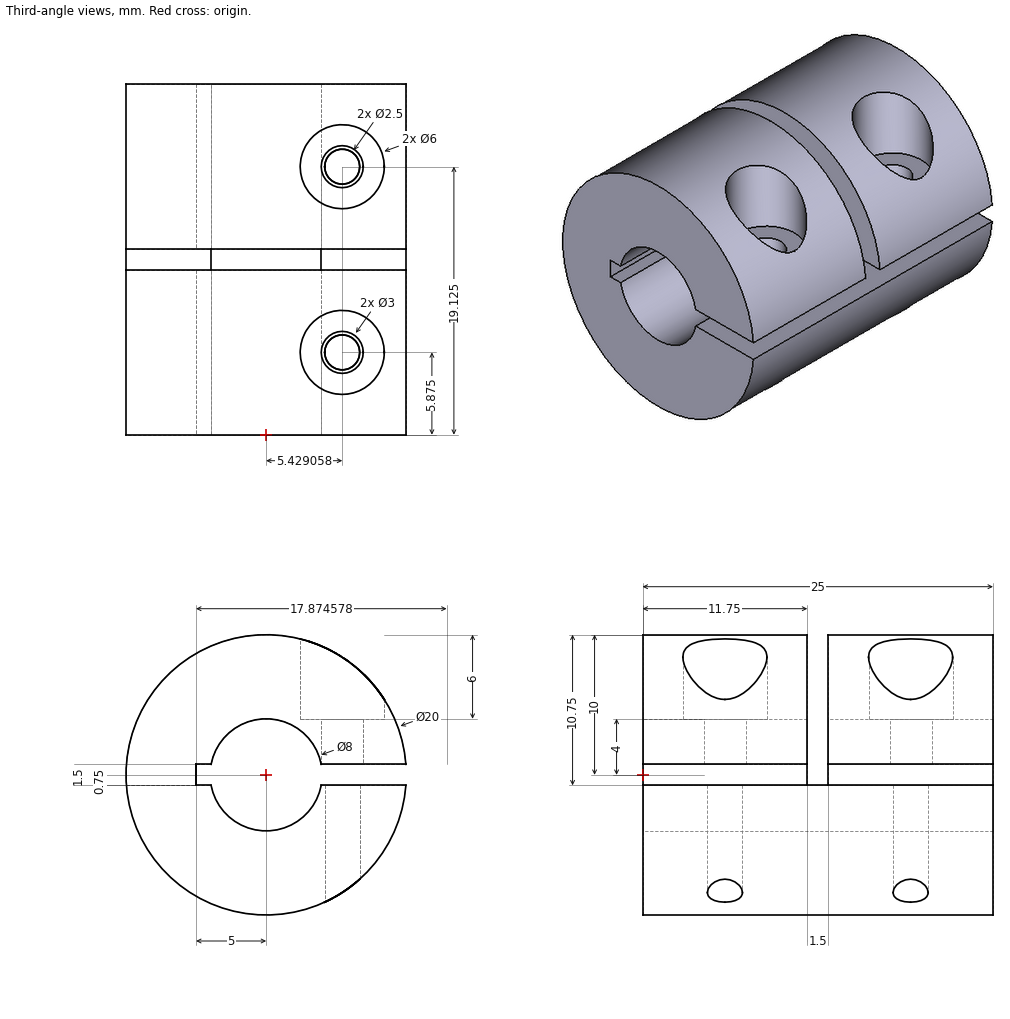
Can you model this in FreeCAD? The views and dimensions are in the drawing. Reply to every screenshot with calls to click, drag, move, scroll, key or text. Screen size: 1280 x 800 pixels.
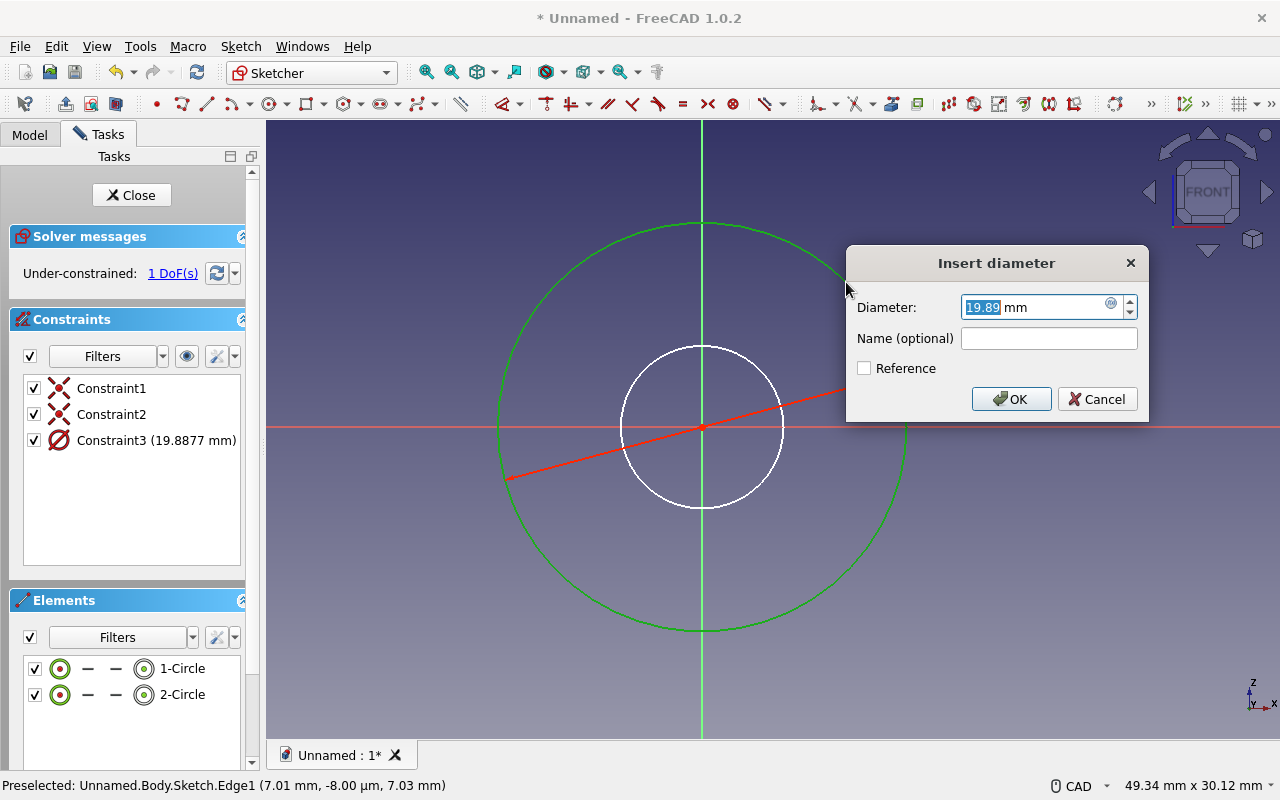
text(20)
key(Return)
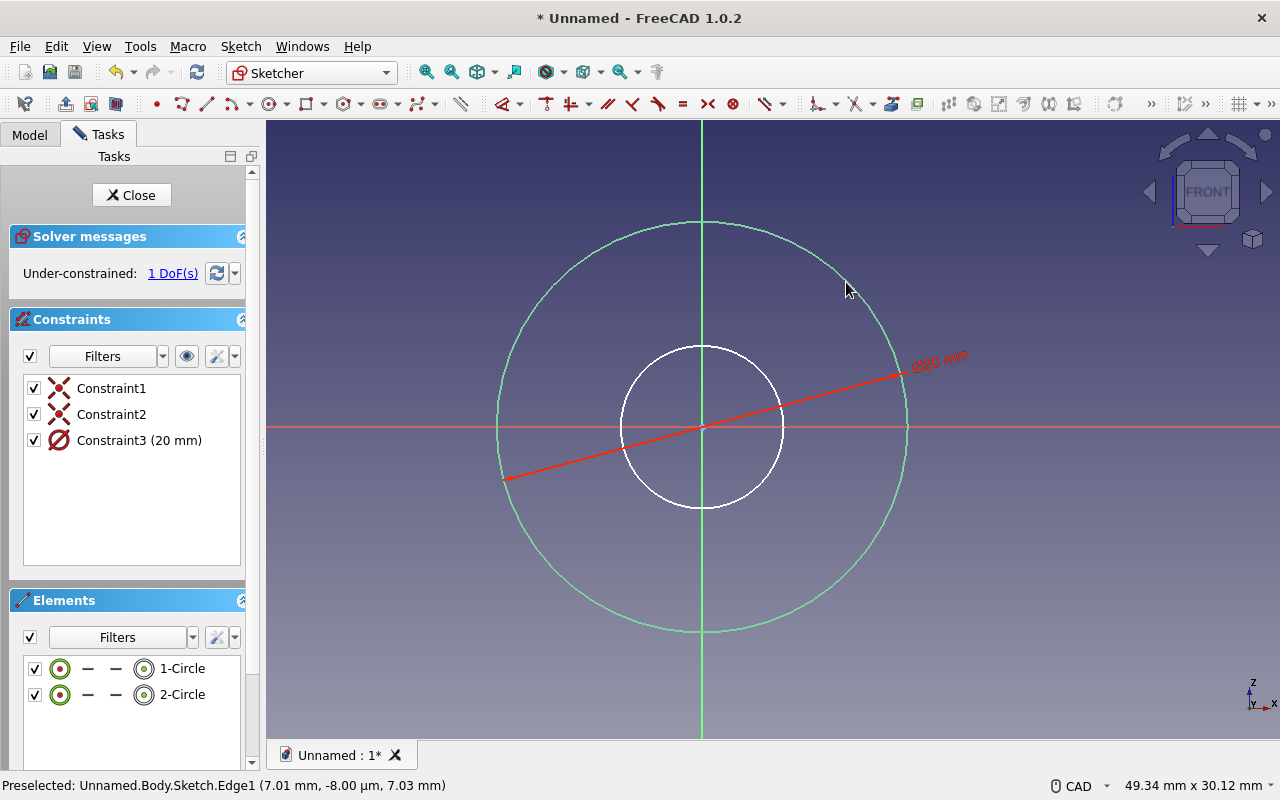
click(759, 369)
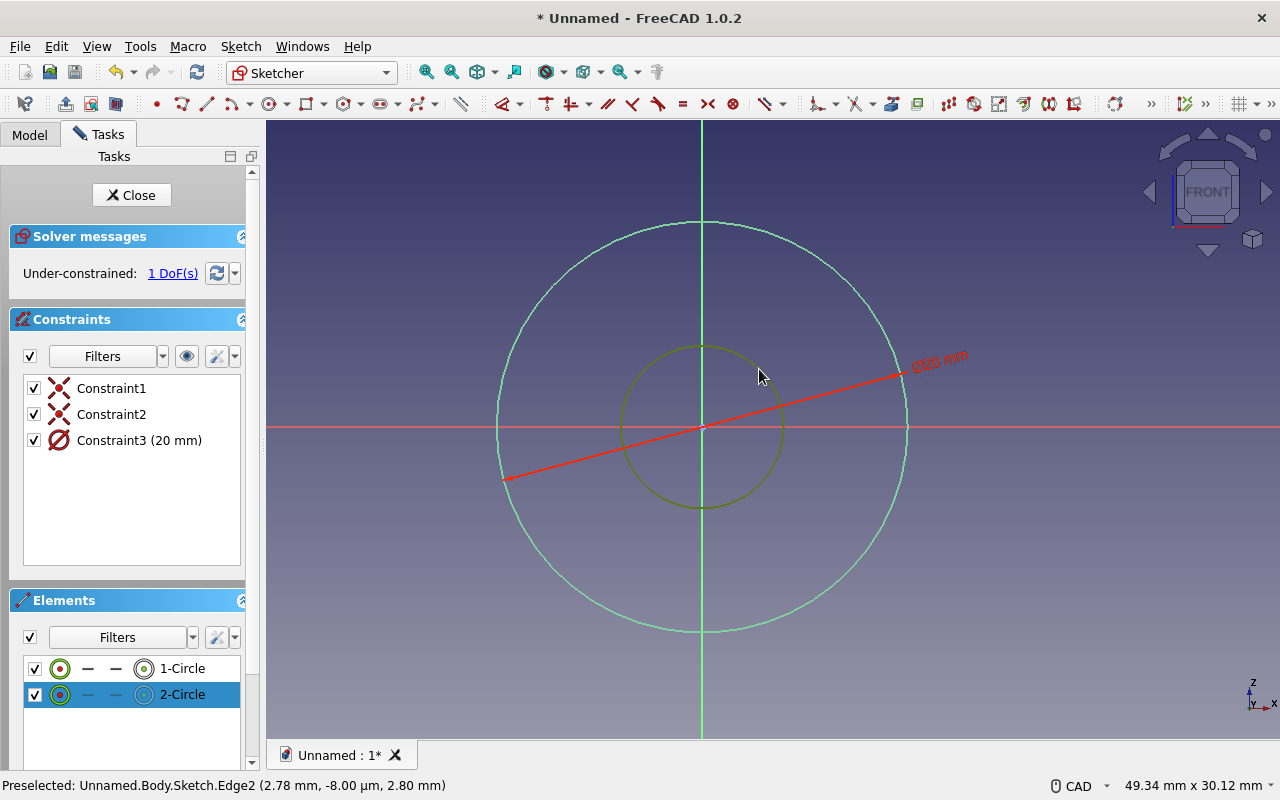
key(k)
key(o)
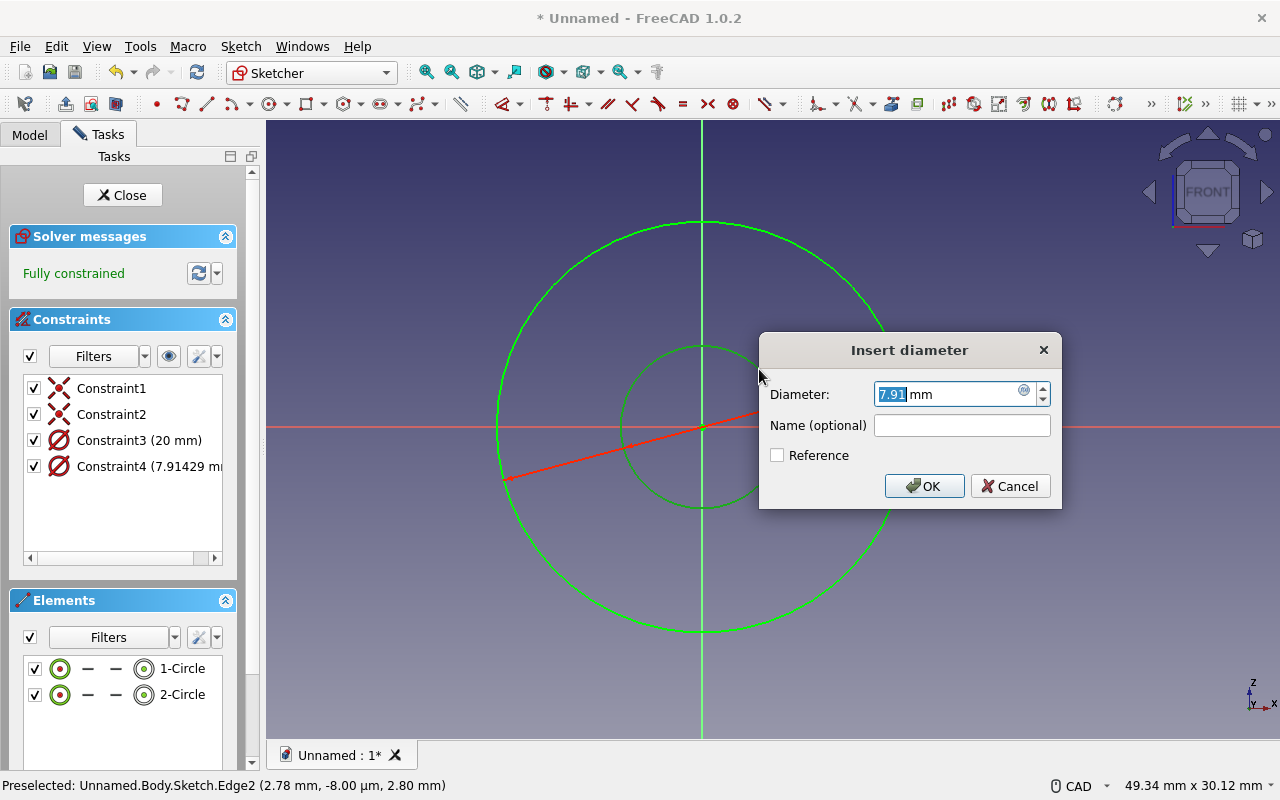
text(8)
key(Return)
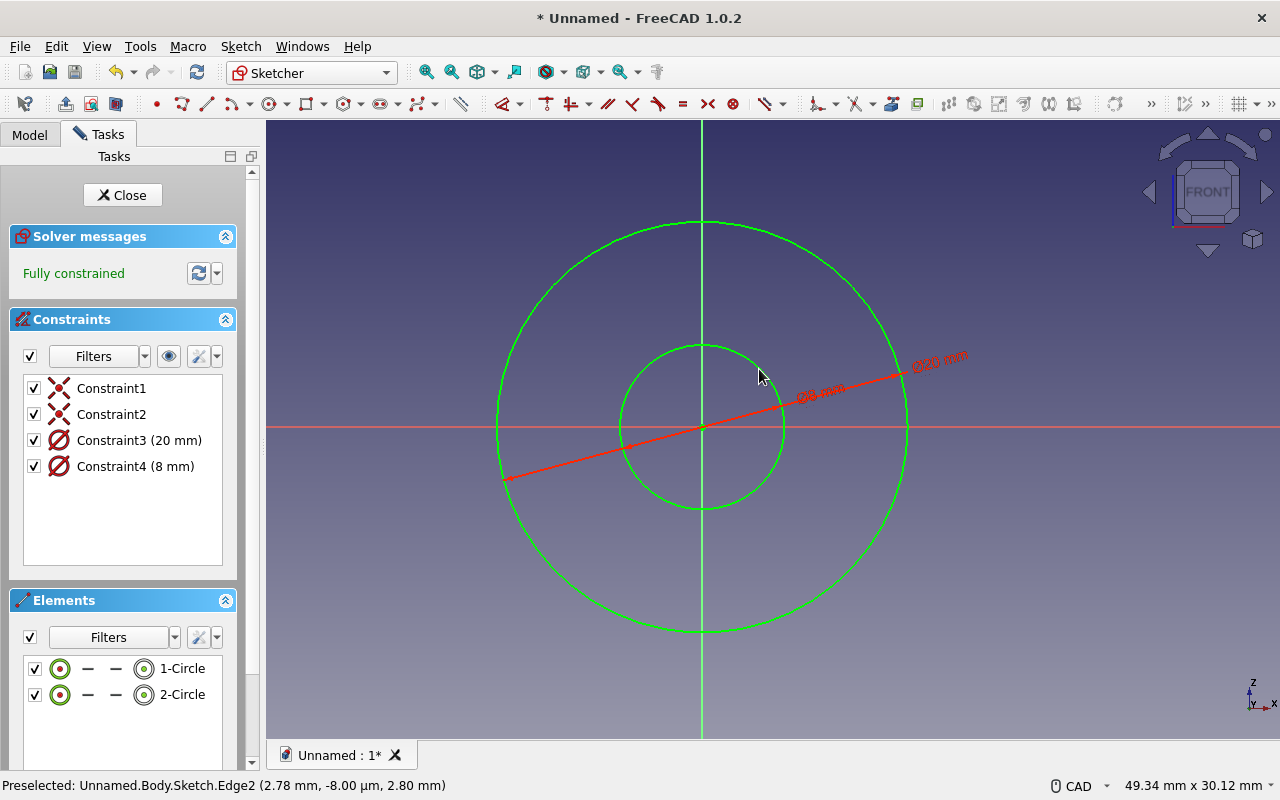
click(123, 195)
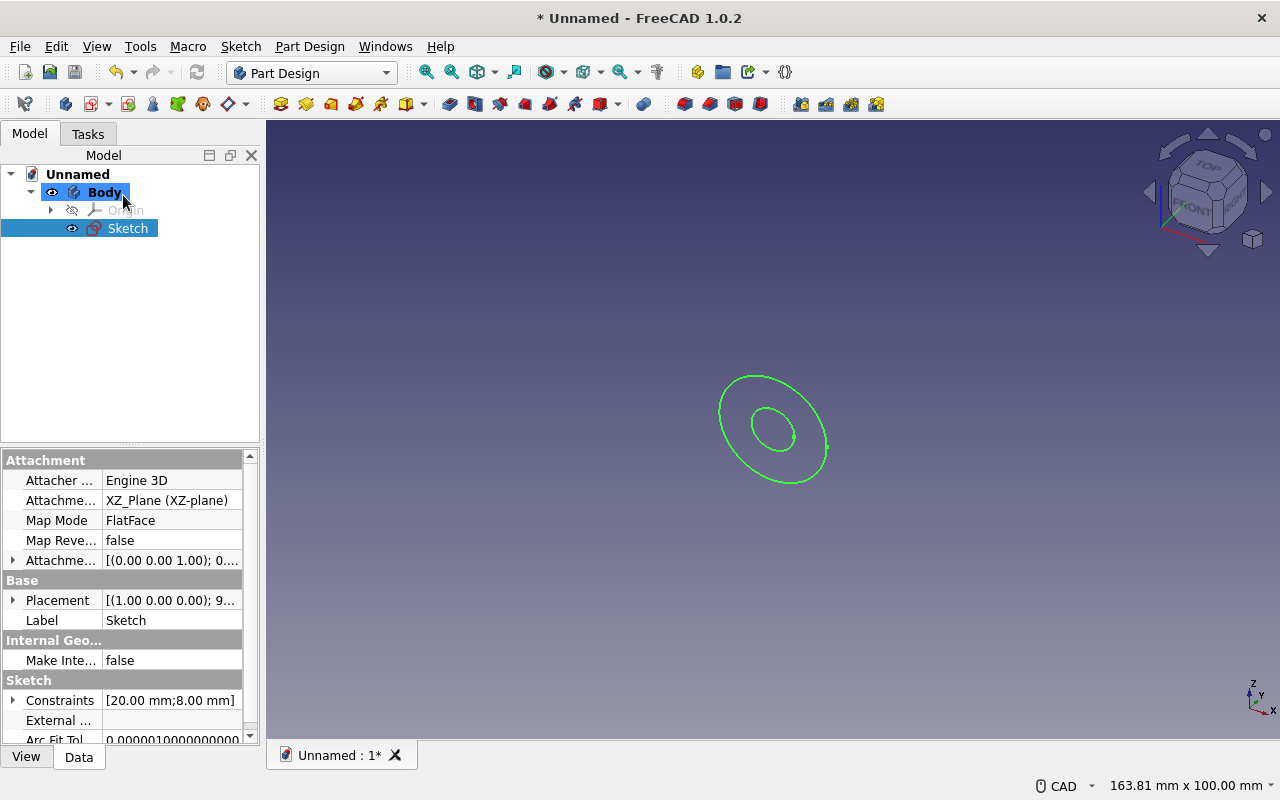
click(281, 104)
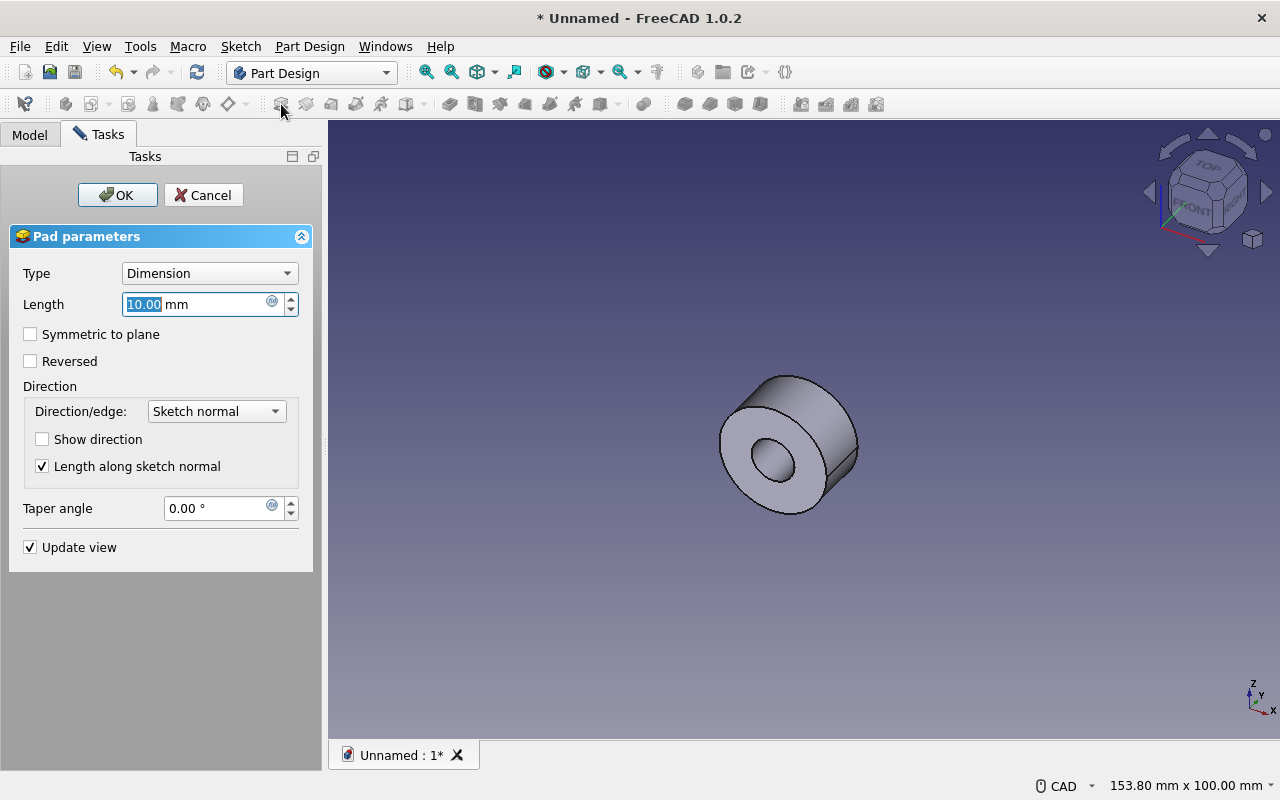
text(25)
key(Tab)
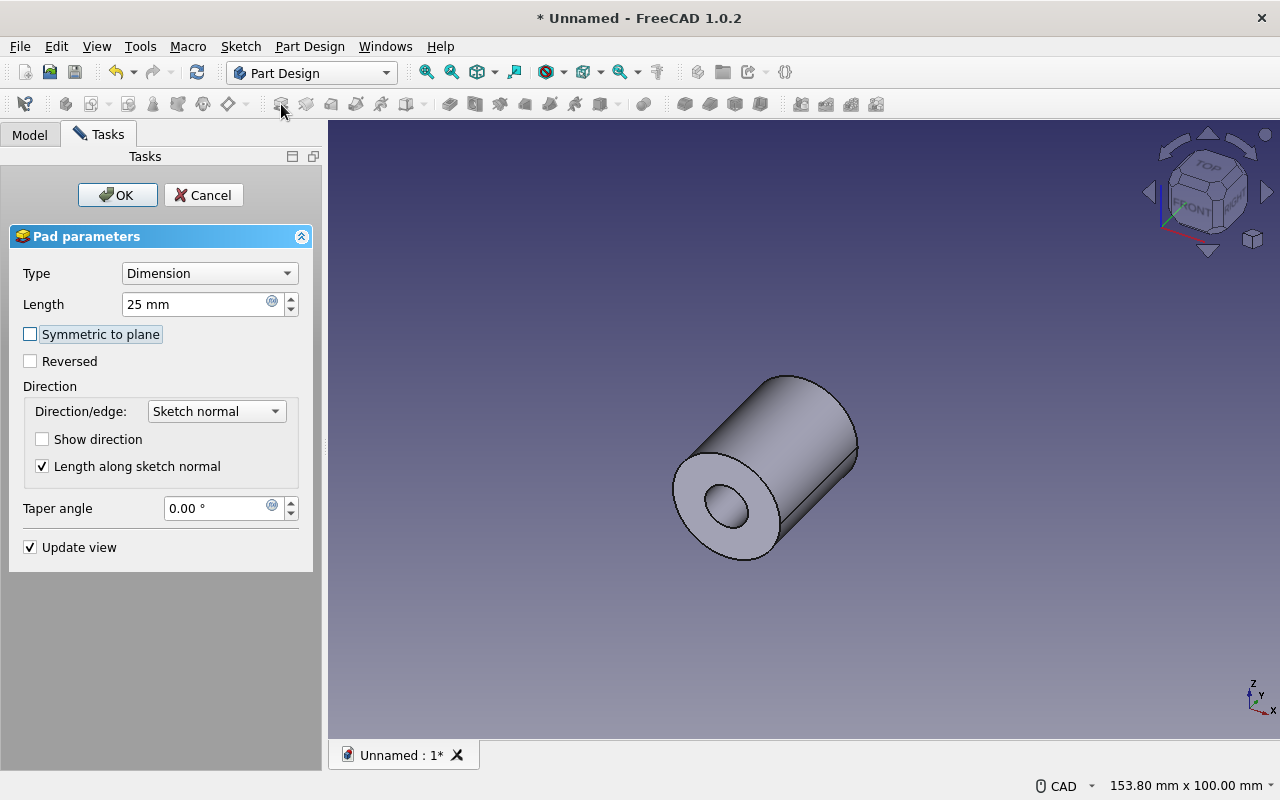
click(31, 361)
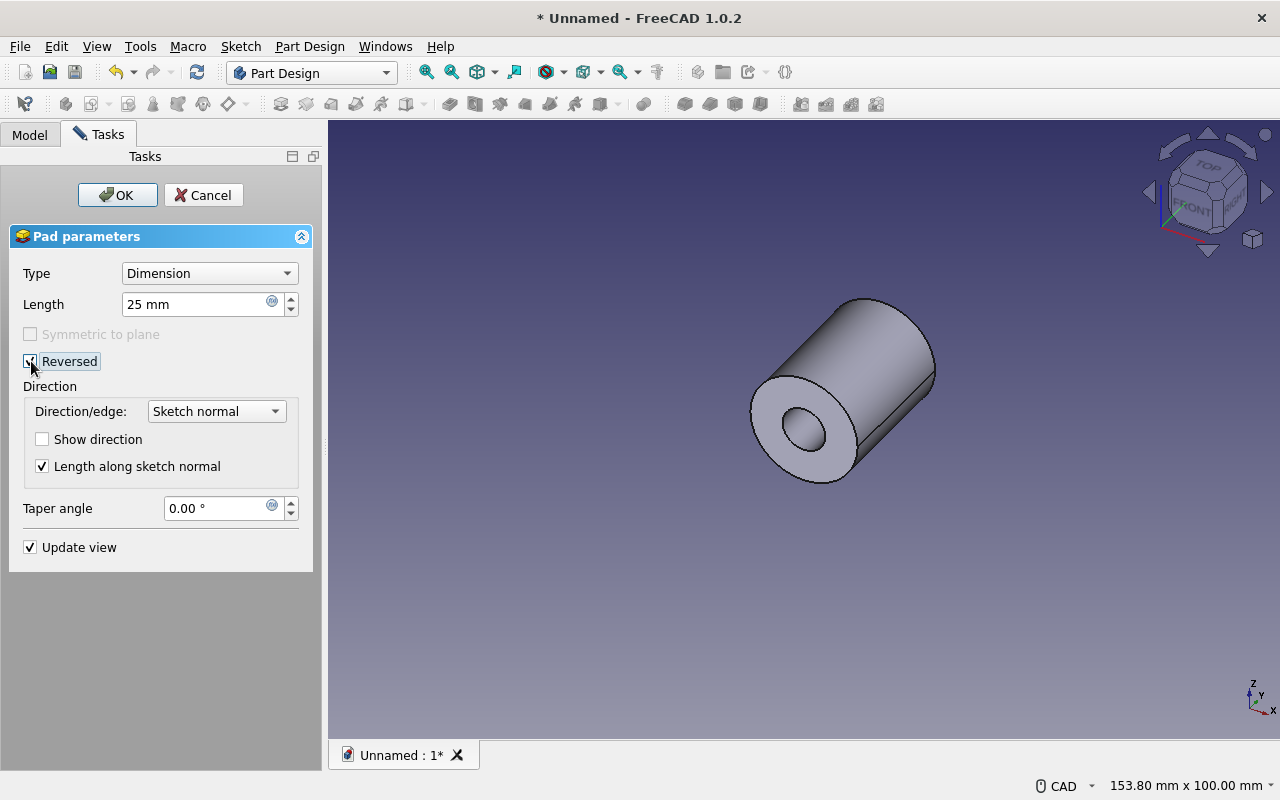
click(118, 195)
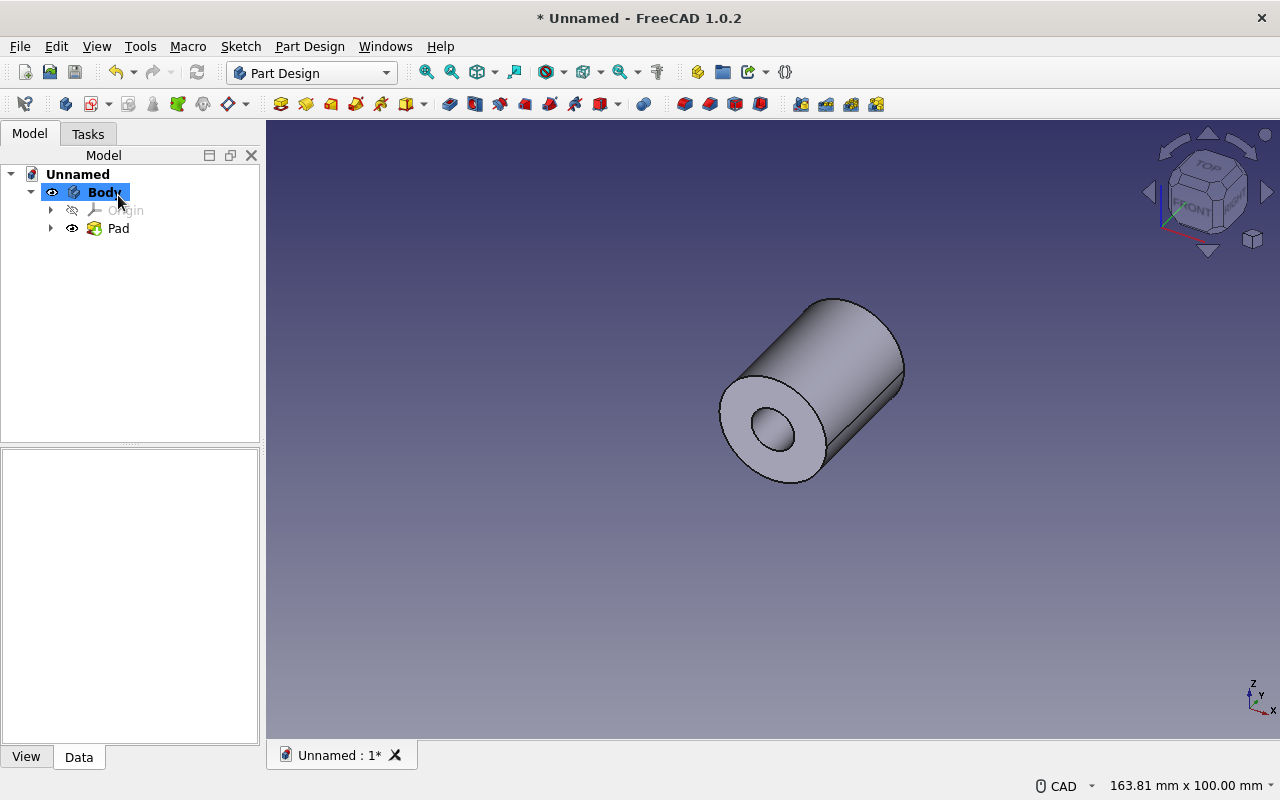
click(427, 72)